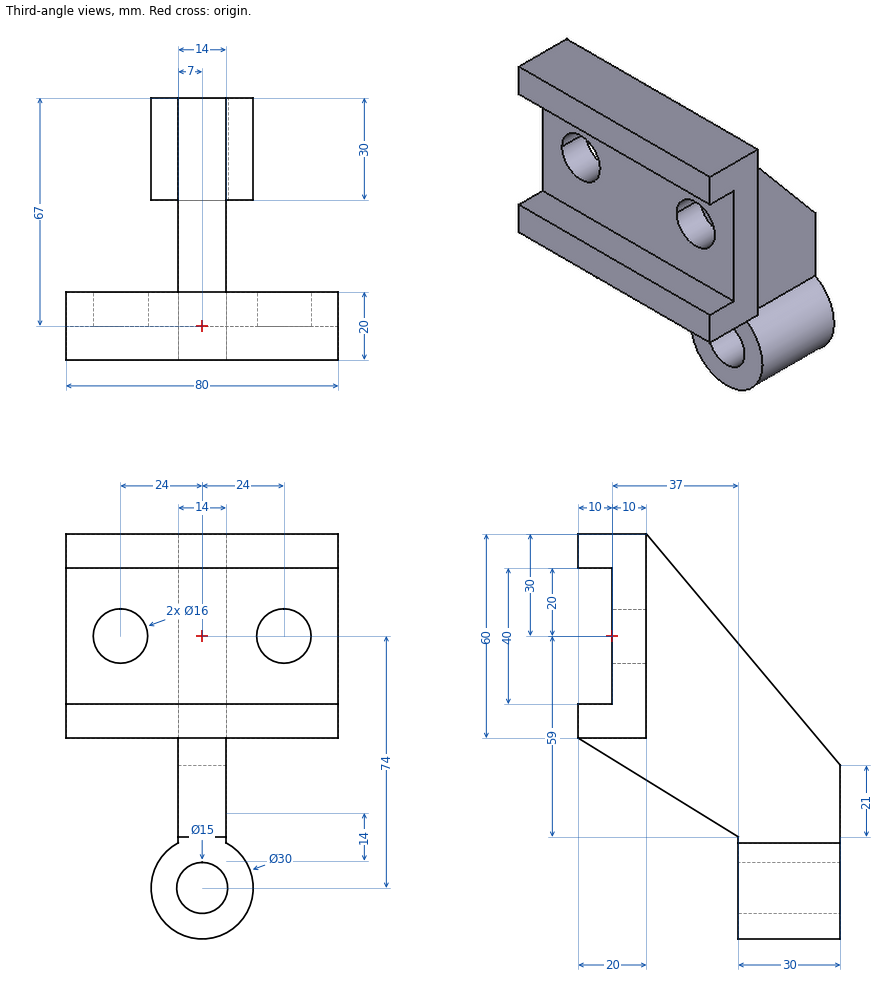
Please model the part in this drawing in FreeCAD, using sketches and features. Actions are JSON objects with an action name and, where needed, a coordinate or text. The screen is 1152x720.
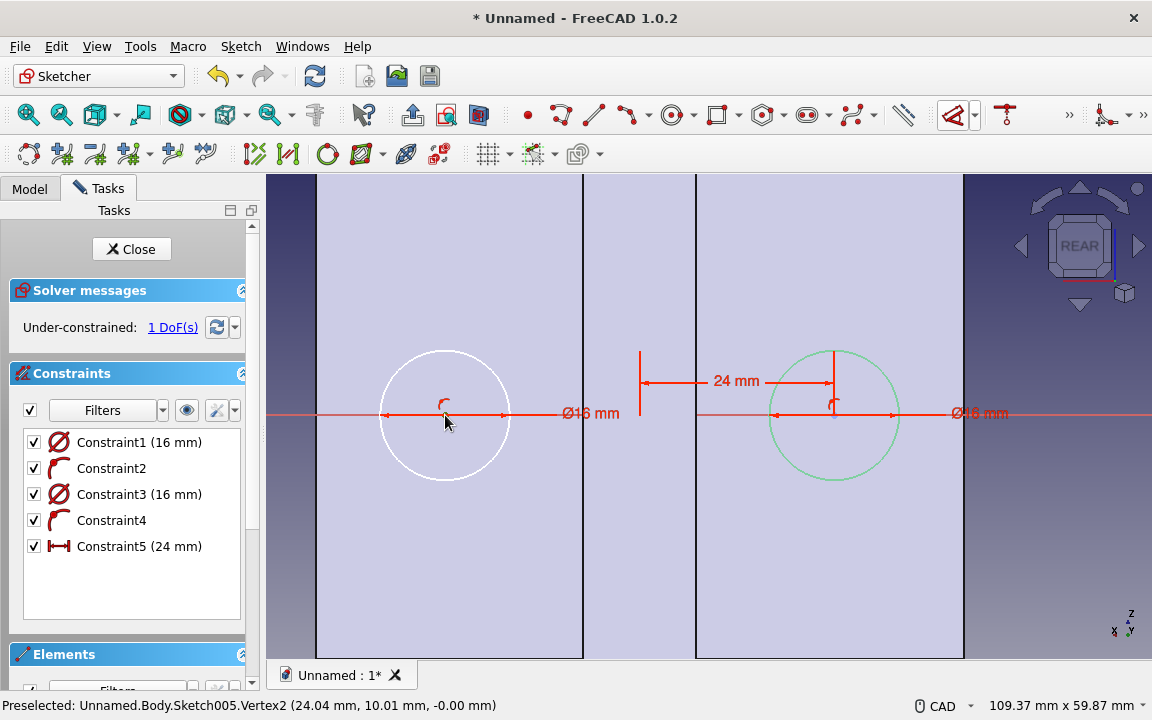
{"action": "left_click", "coordinate": [974, 116]}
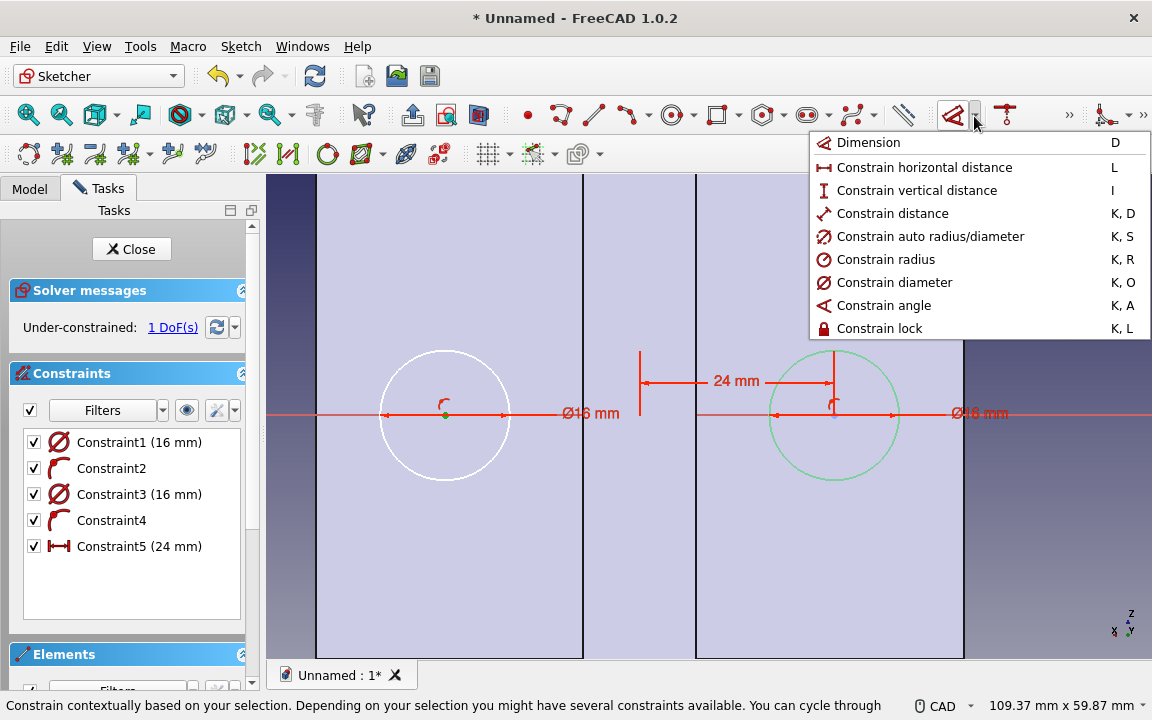
{"action": "left_click", "coordinate": [980, 168]}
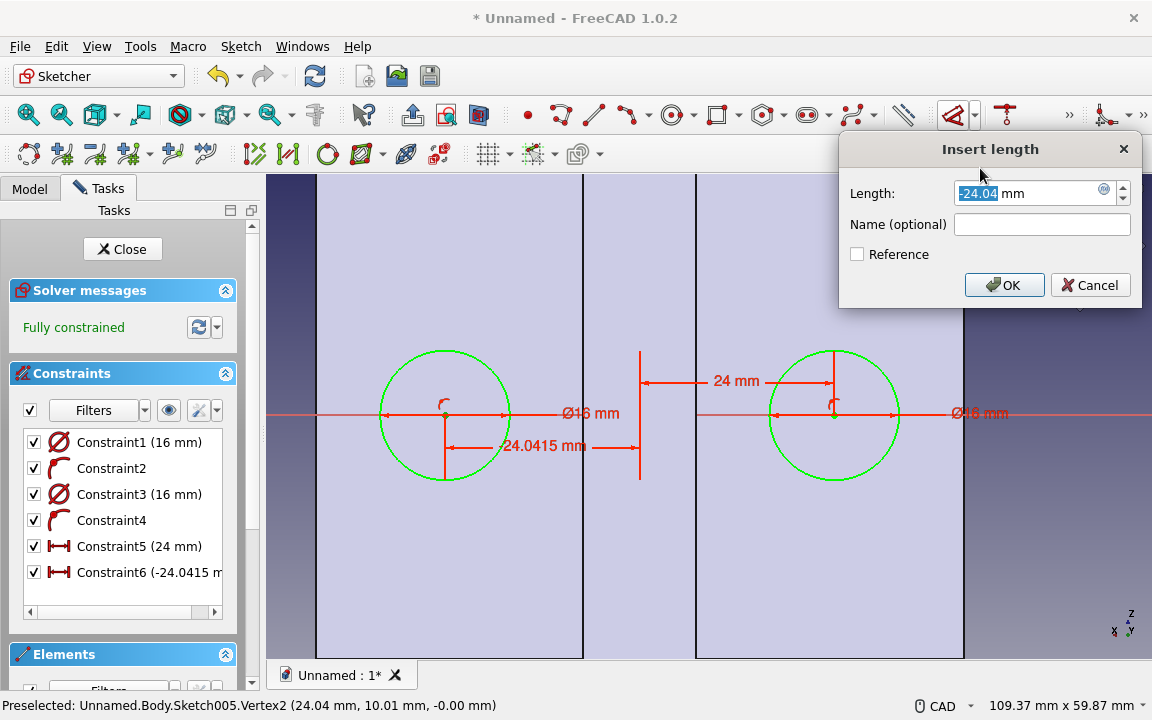
{"action": "type", "text": "-24"}
{"action": "key", "text": "Return"}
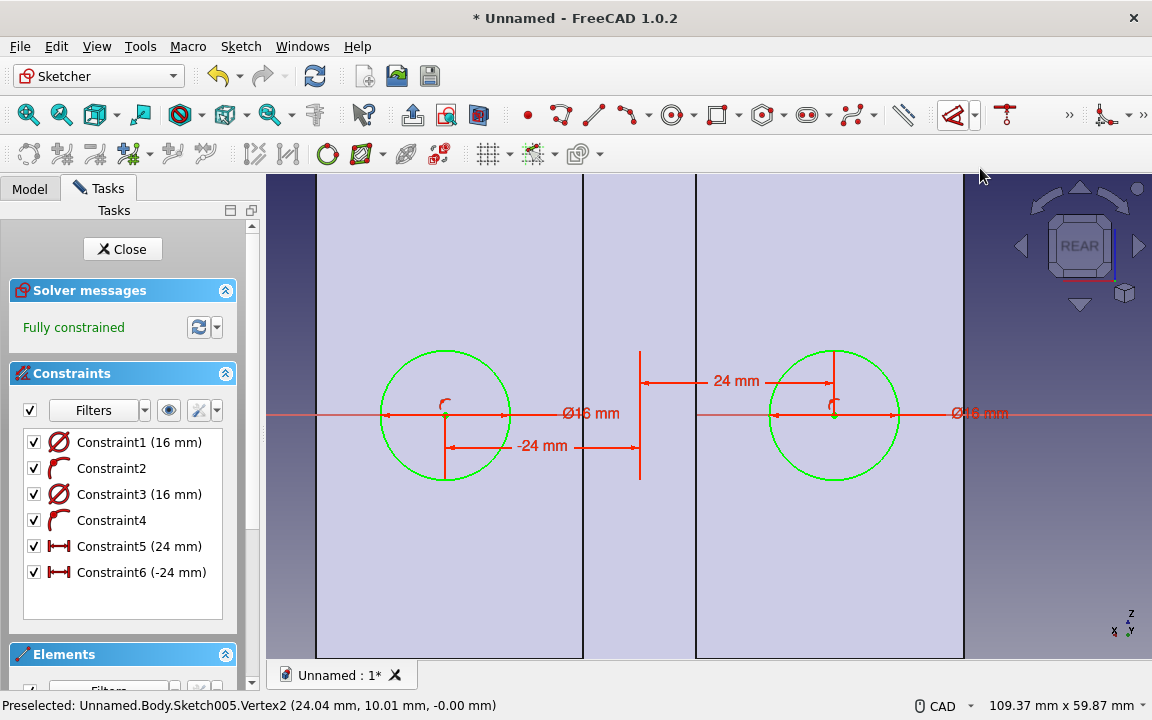
{"action": "left_click", "coordinate": [123, 249]}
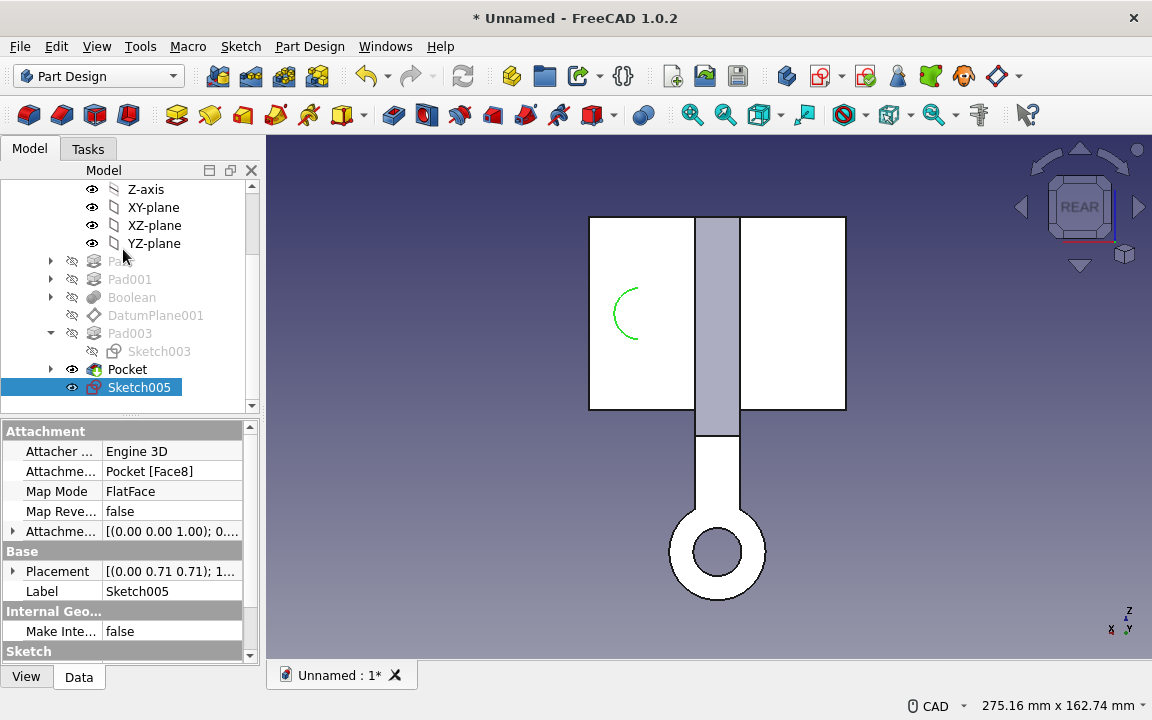
{"action": "left_click", "coordinate": [394, 116]}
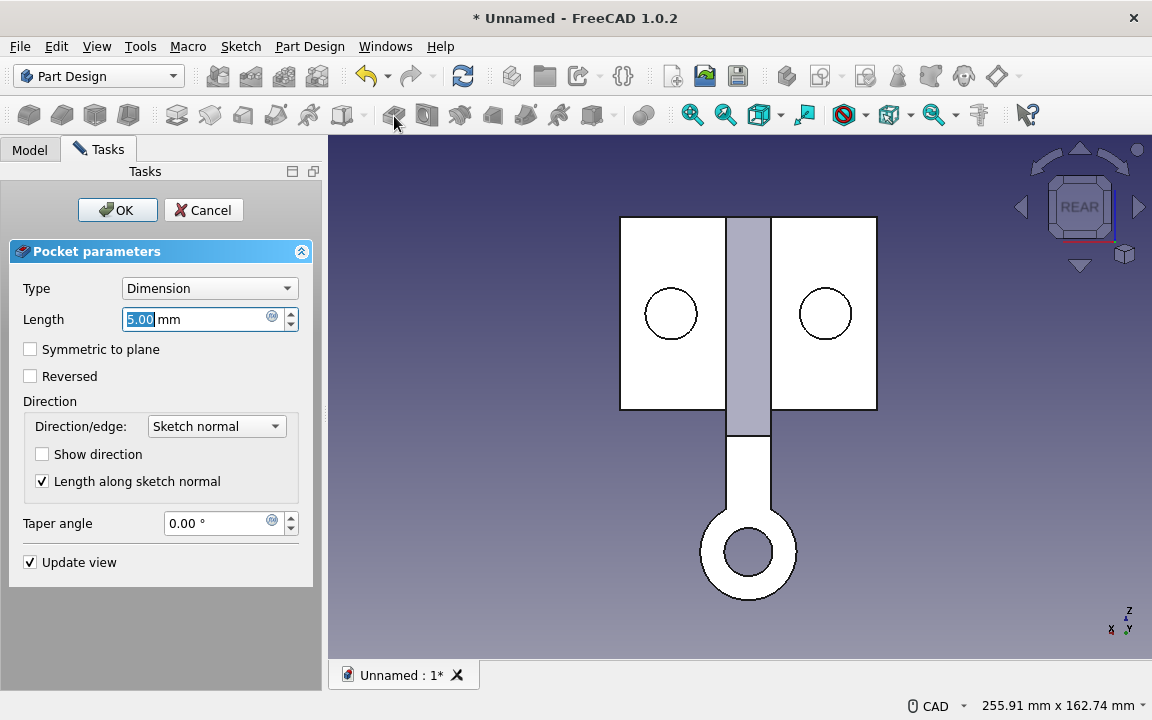
{"action": "left_click", "coordinate": [210, 288]}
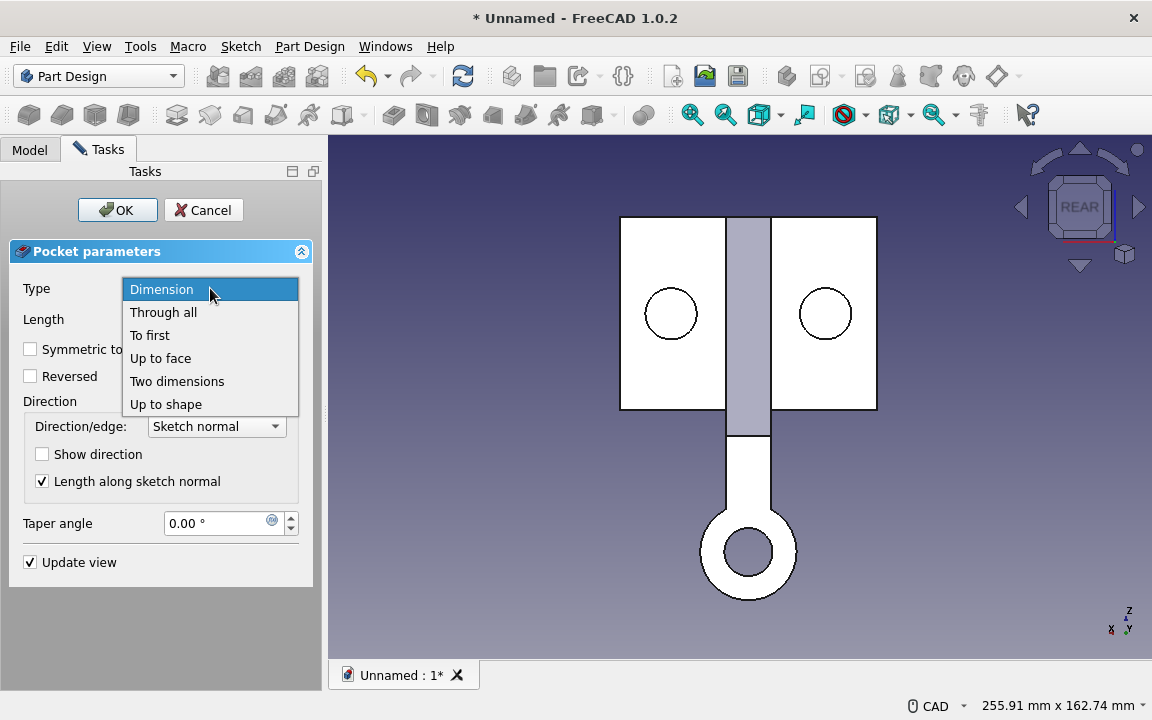
{"action": "left_click", "coordinate": [208, 312]}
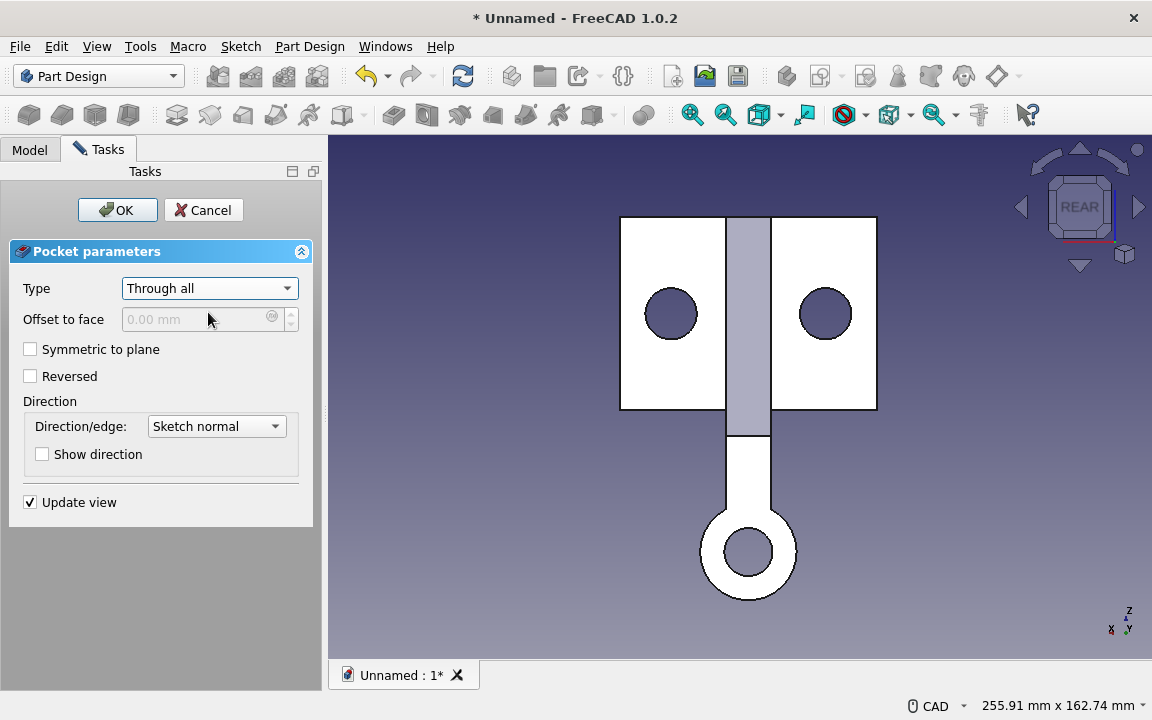
{"action": "left_click", "coordinate": [118, 210]}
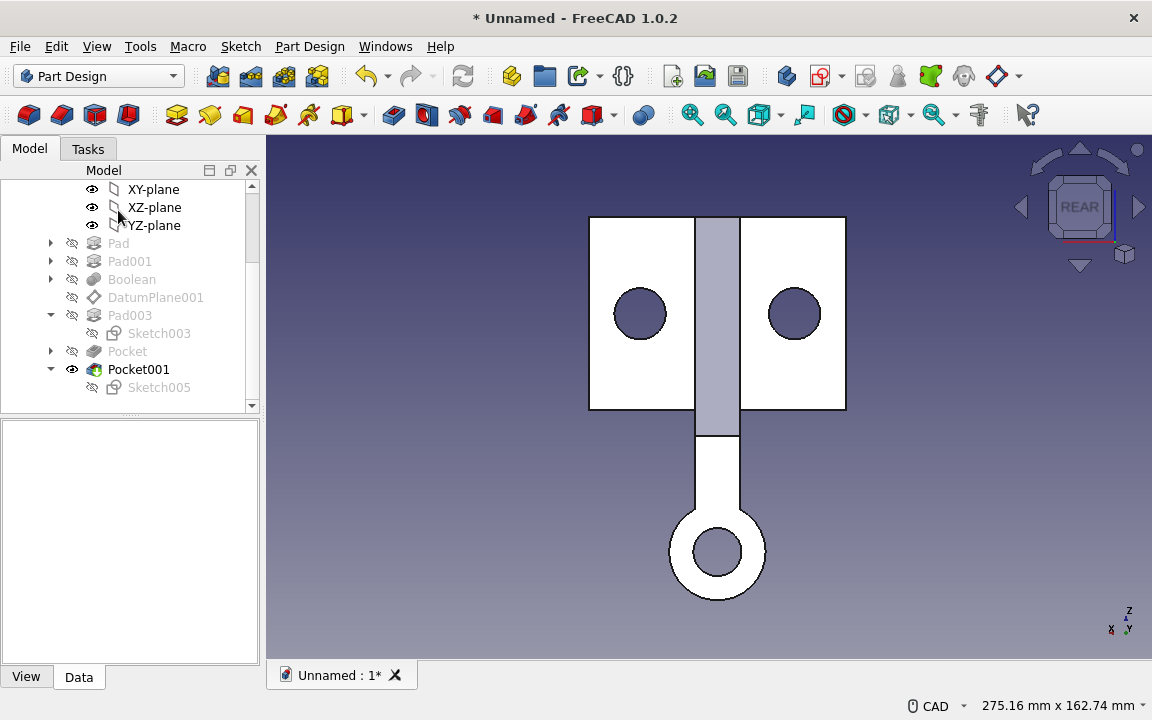
{"action": "key", "text": "0"}